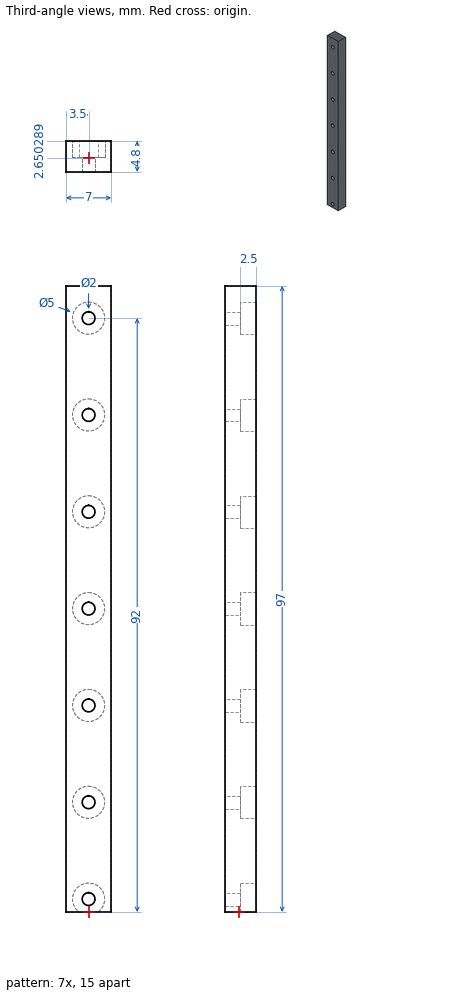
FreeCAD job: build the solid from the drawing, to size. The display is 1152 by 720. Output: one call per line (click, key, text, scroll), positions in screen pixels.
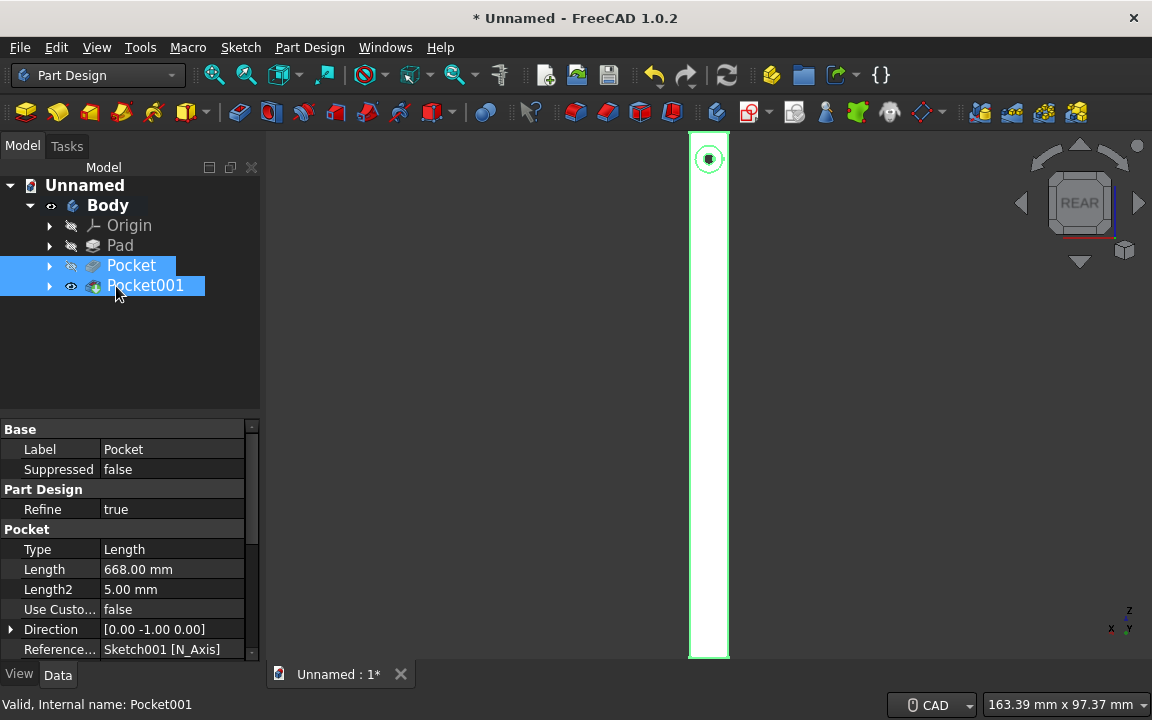
click(1012, 112)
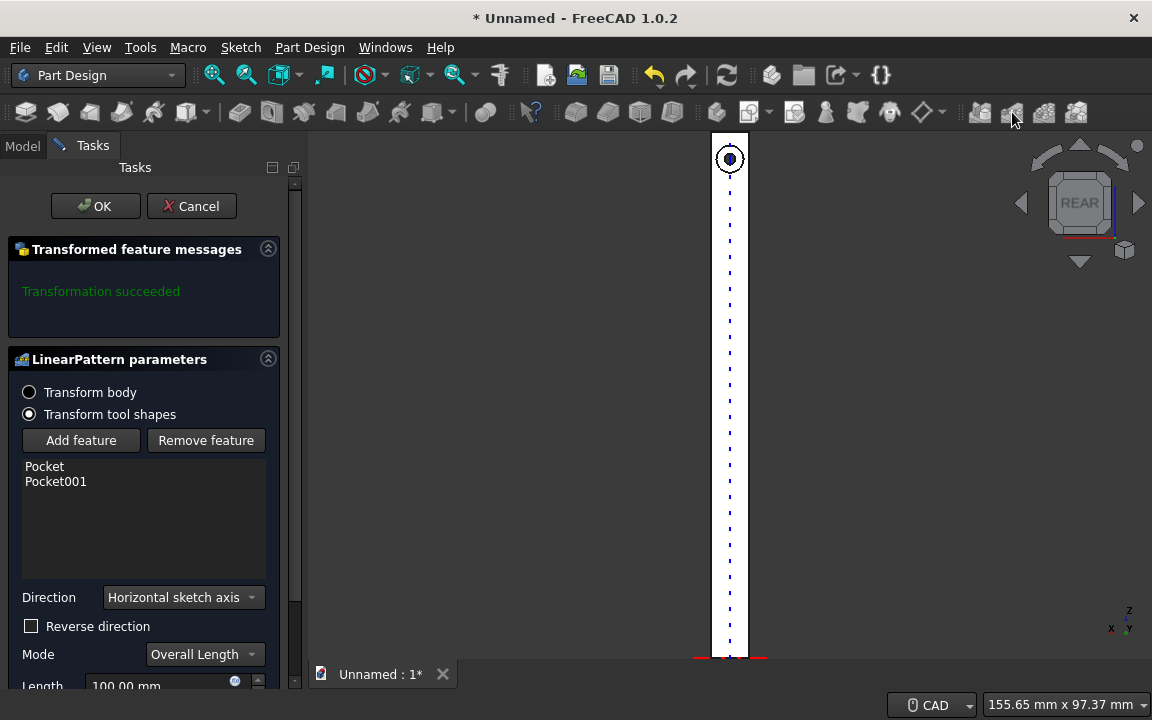
click(184, 598)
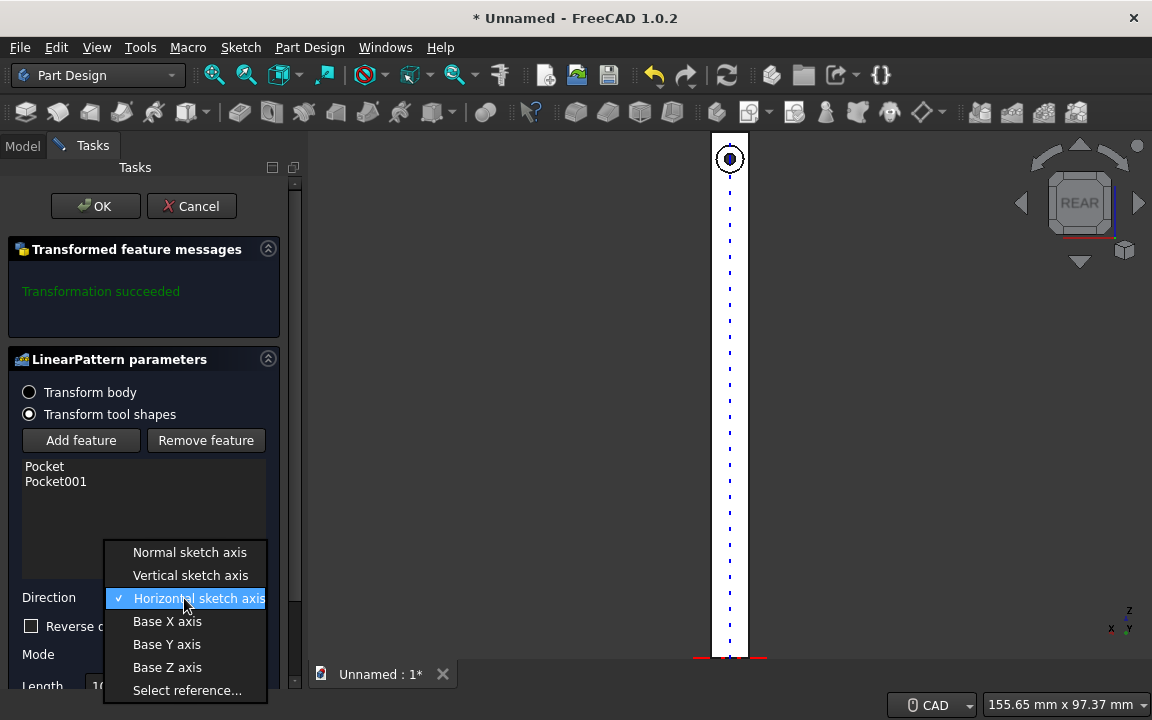
click(184, 668)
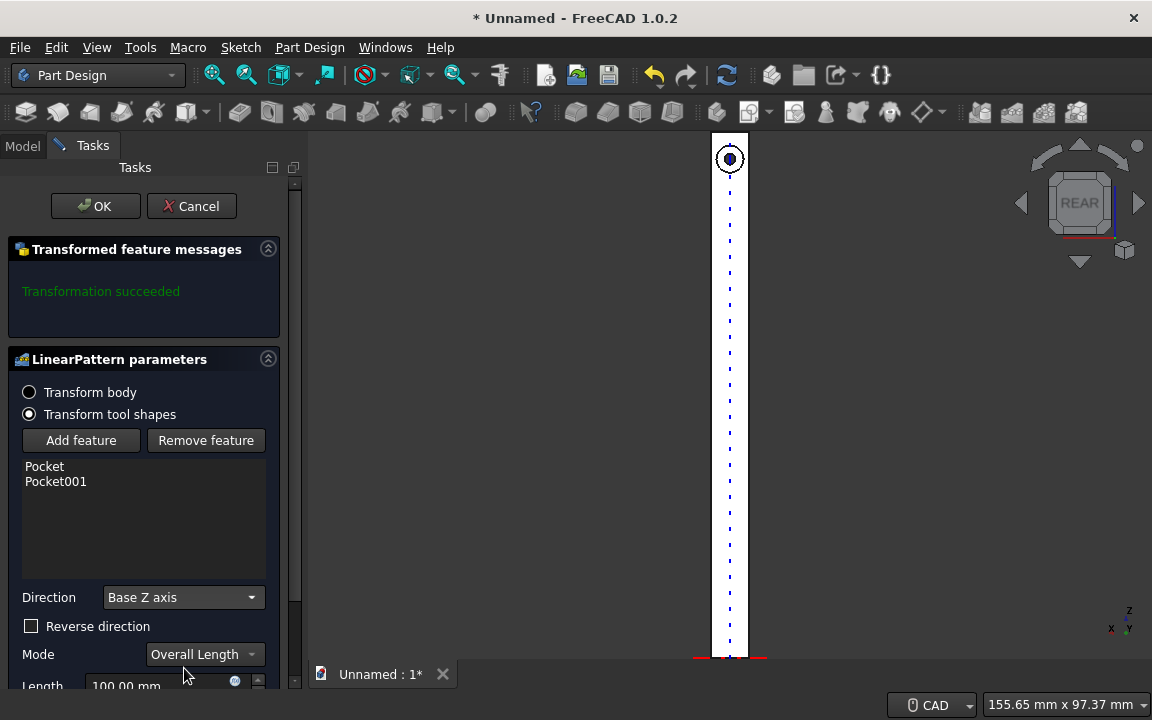
click(206, 654)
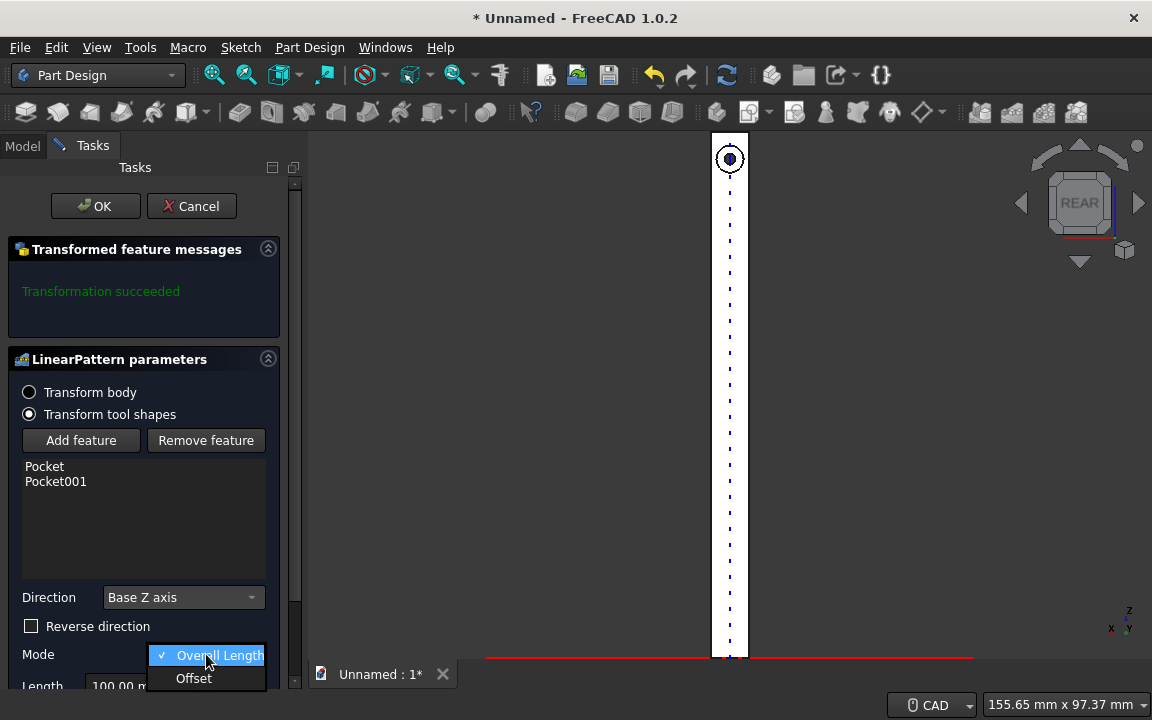
click(206, 678)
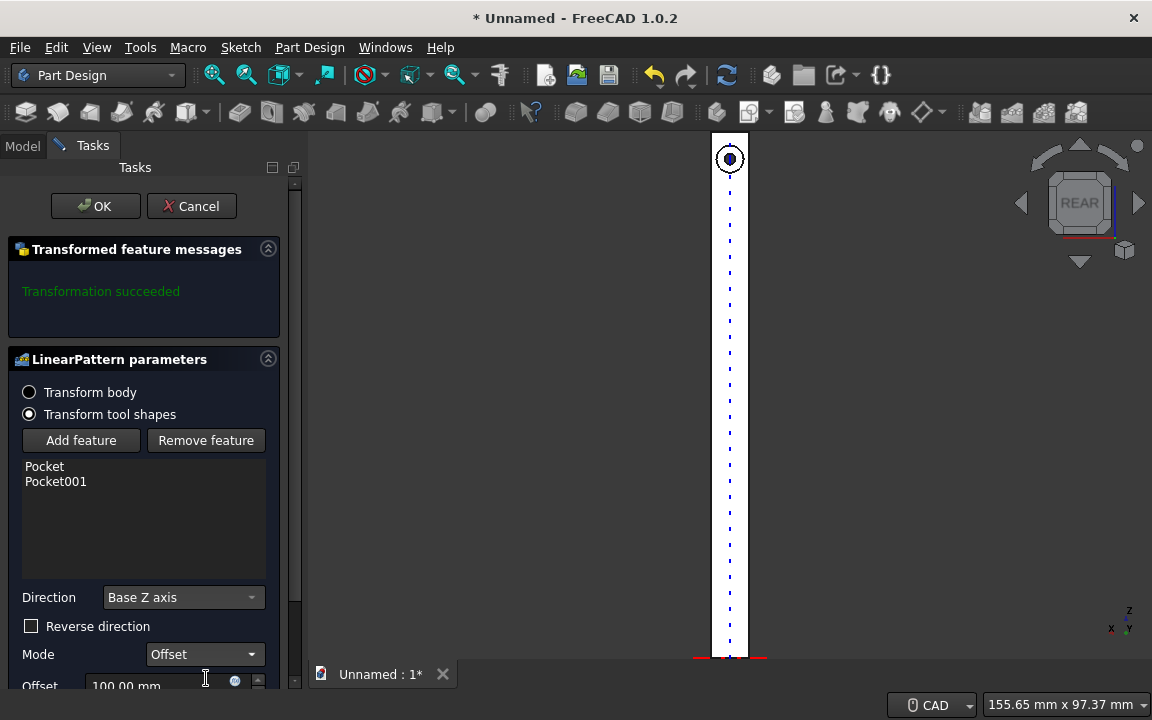
scroll(295, 432, down, 2)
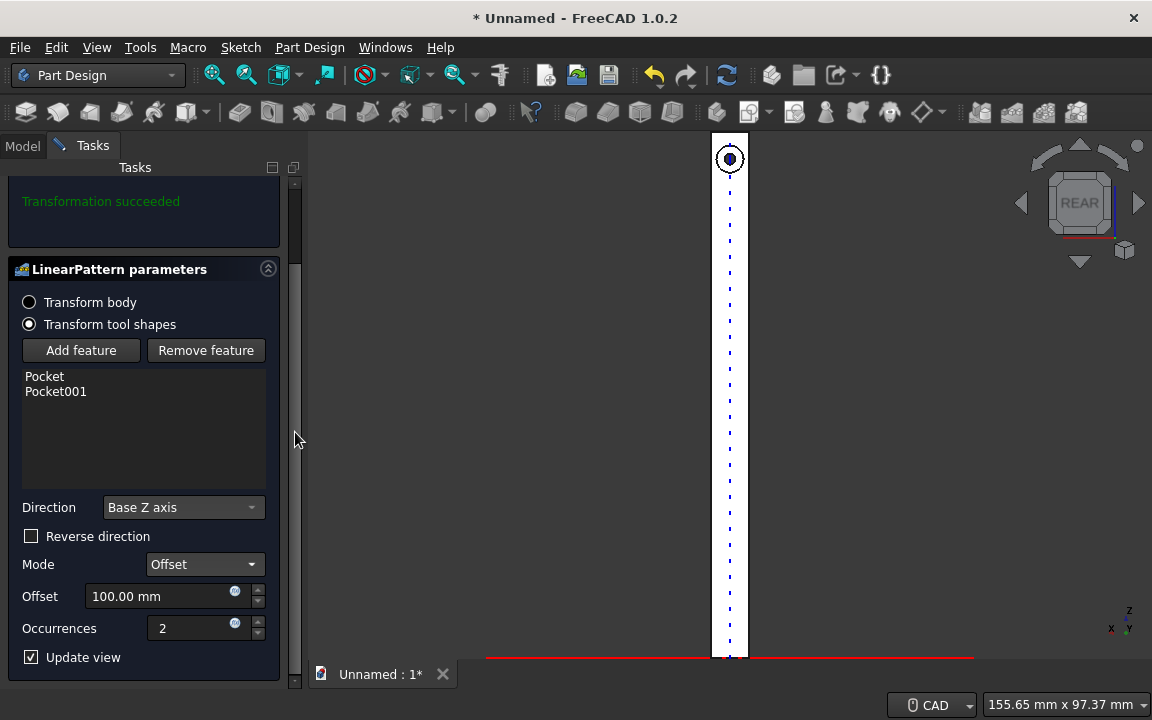
triple_click(168, 596)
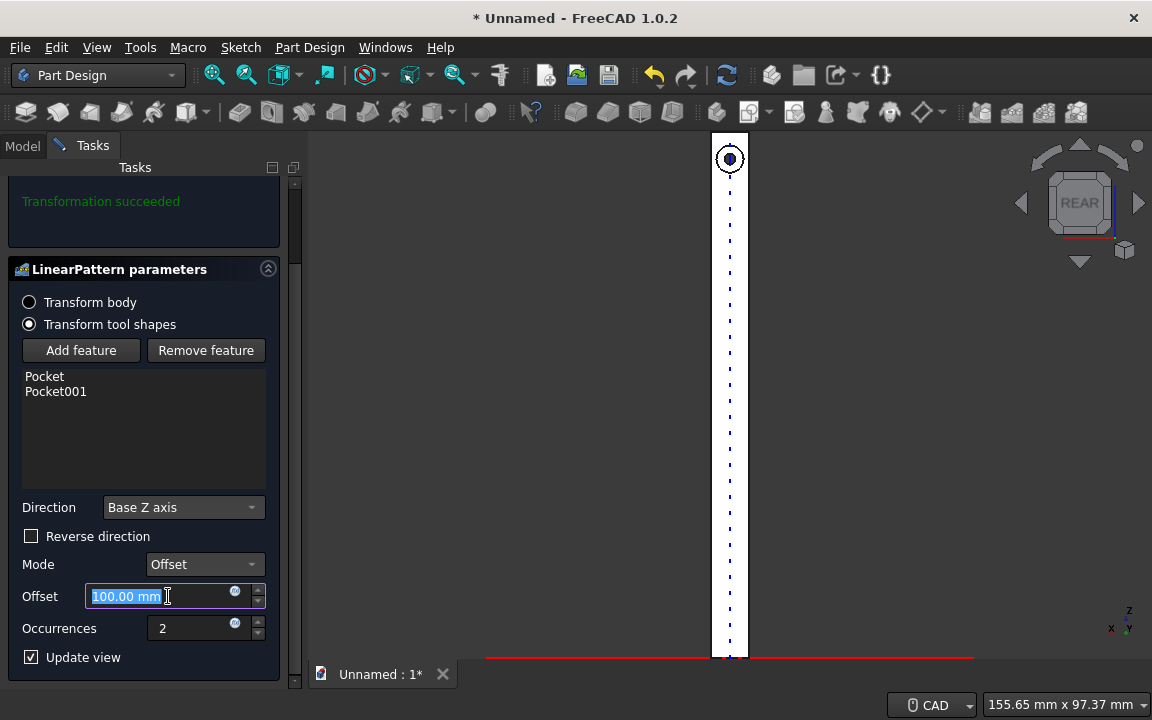
text(15)
key(Tab)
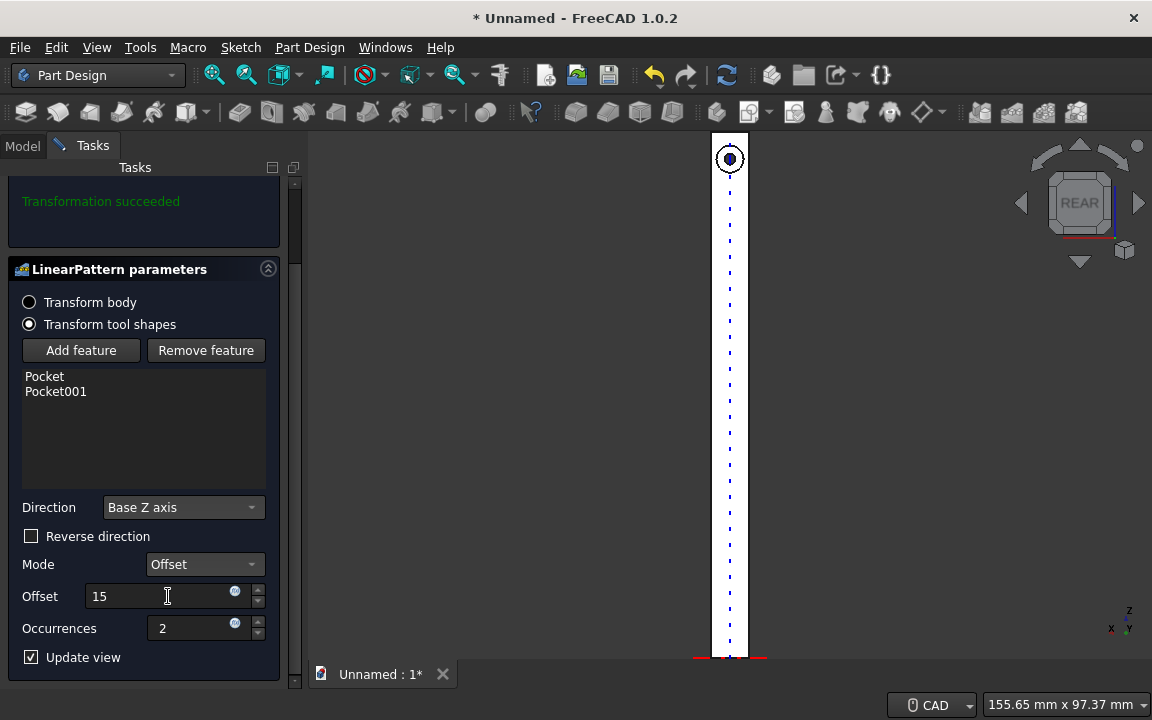
triple_click(198, 628)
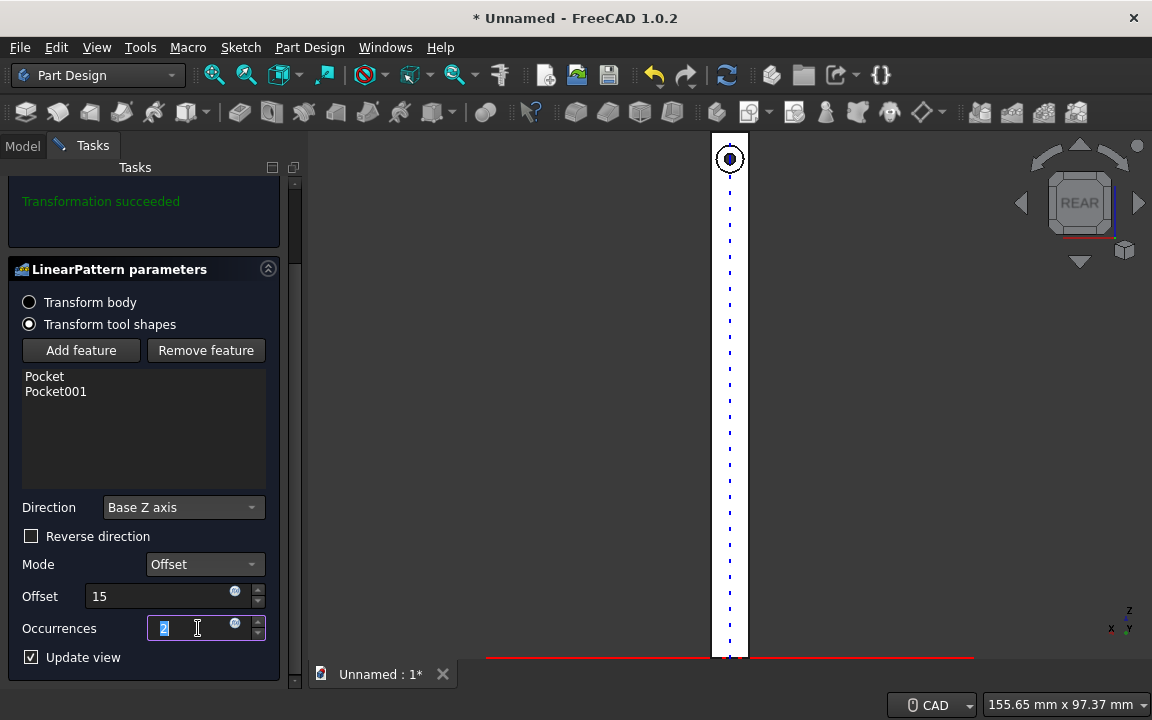
text(7)
key(Tab)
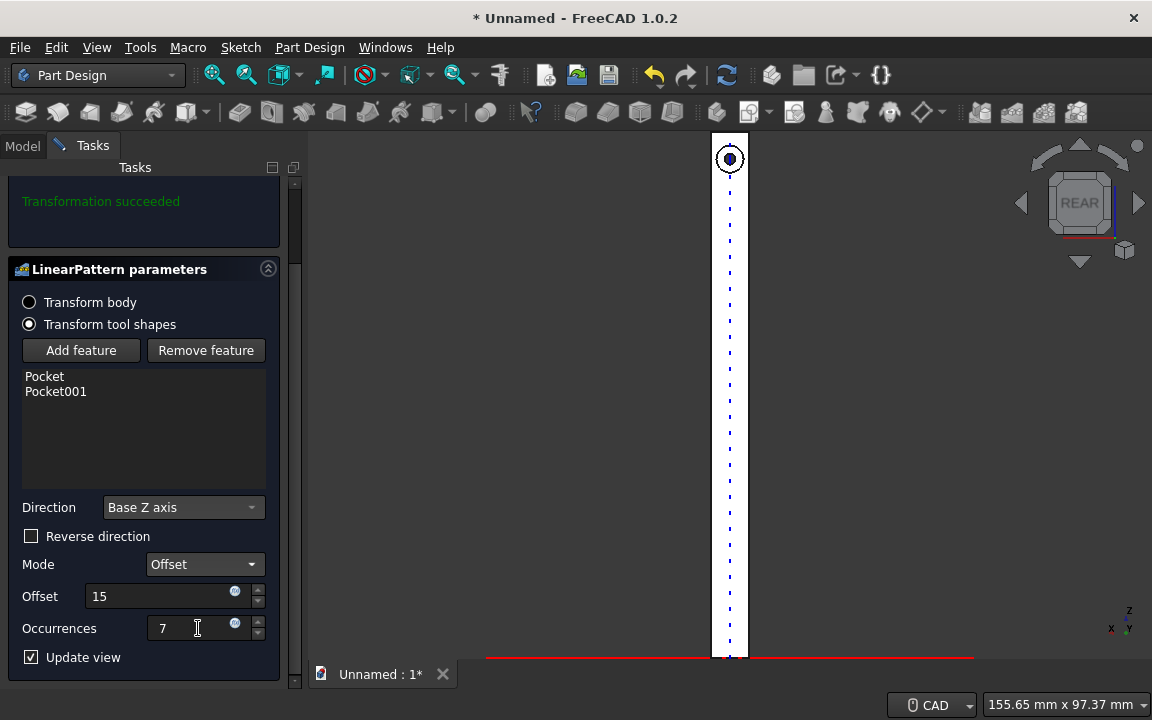
click(30, 536)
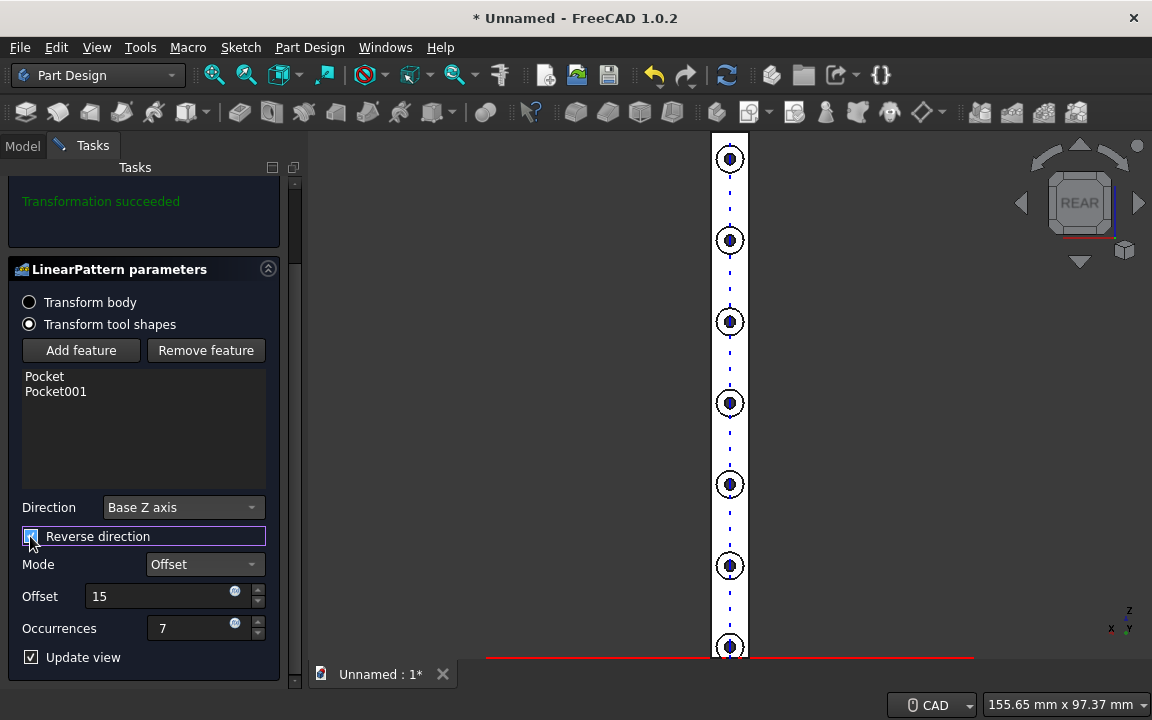
scroll(295, 432, up, 3)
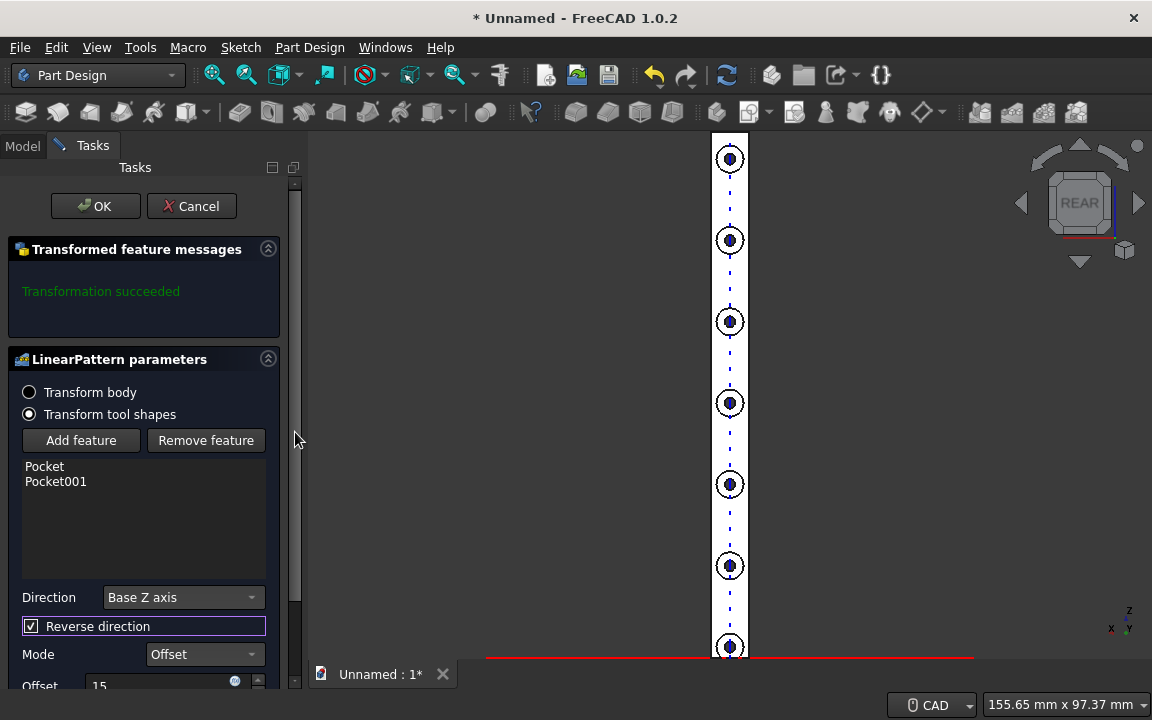
click(96, 206)